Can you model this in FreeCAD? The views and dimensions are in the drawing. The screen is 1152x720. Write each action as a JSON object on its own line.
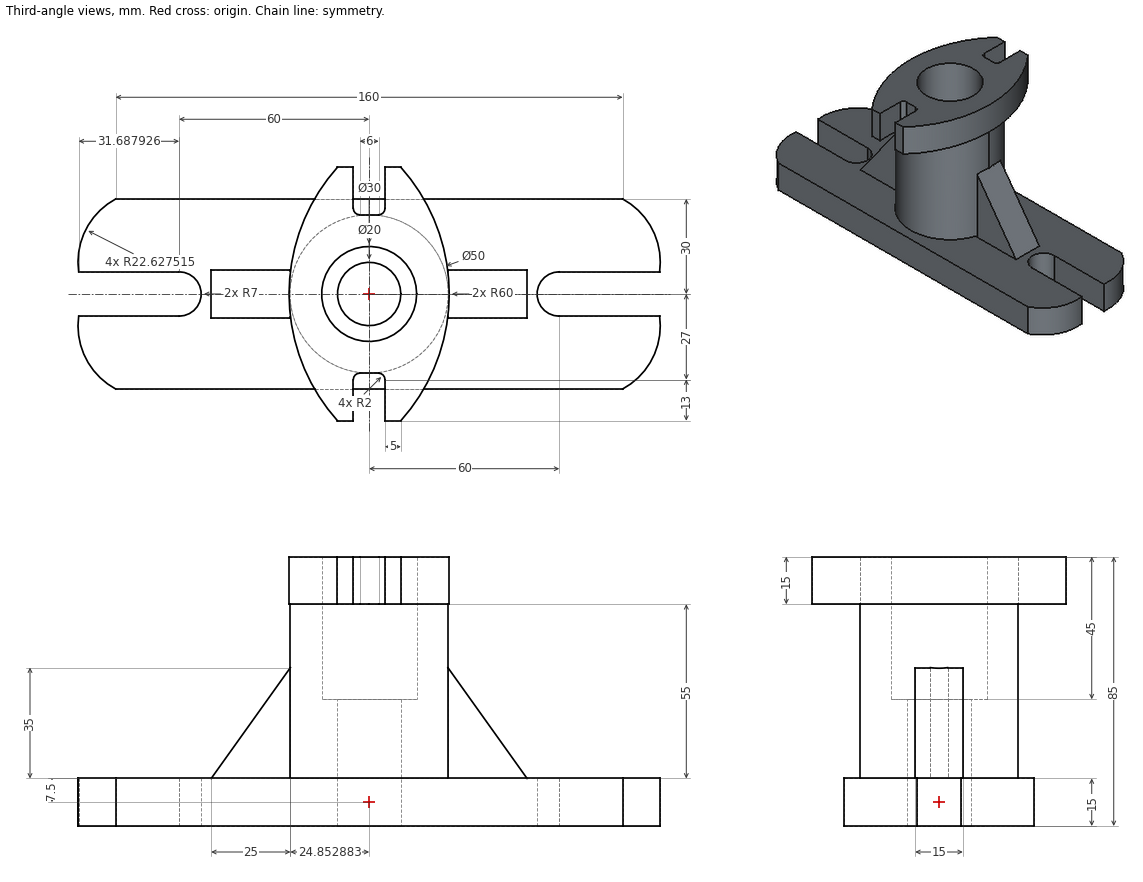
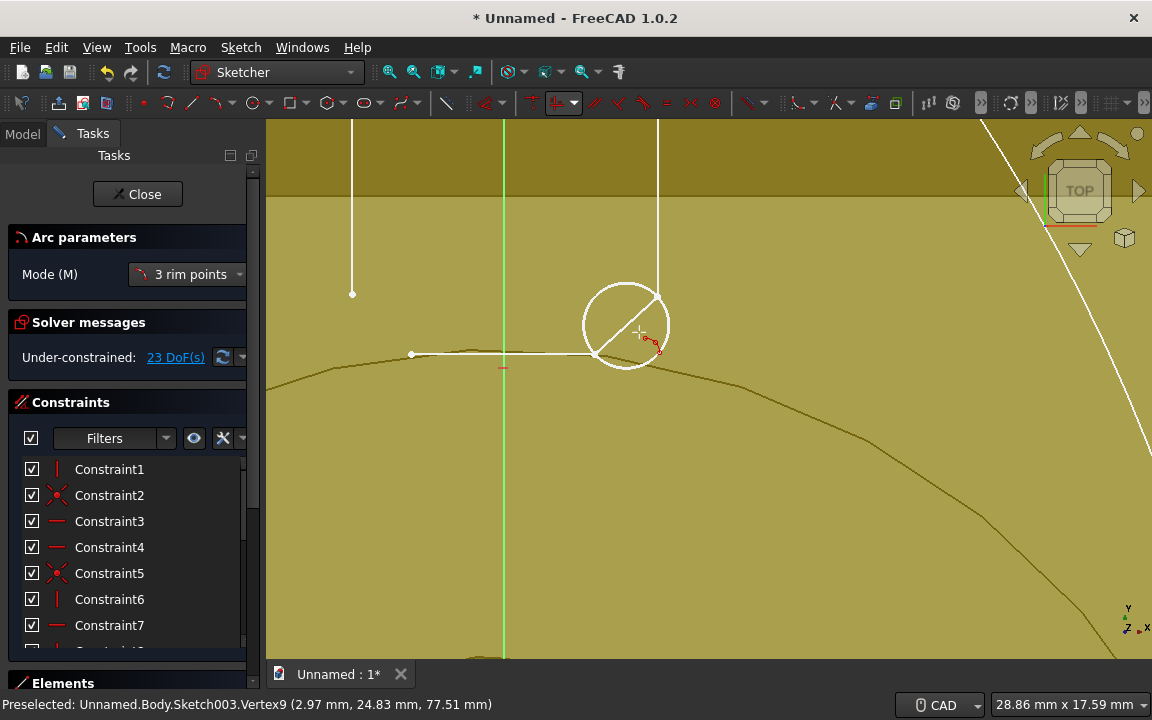
{"action": "left_click", "coordinate": [639, 331]}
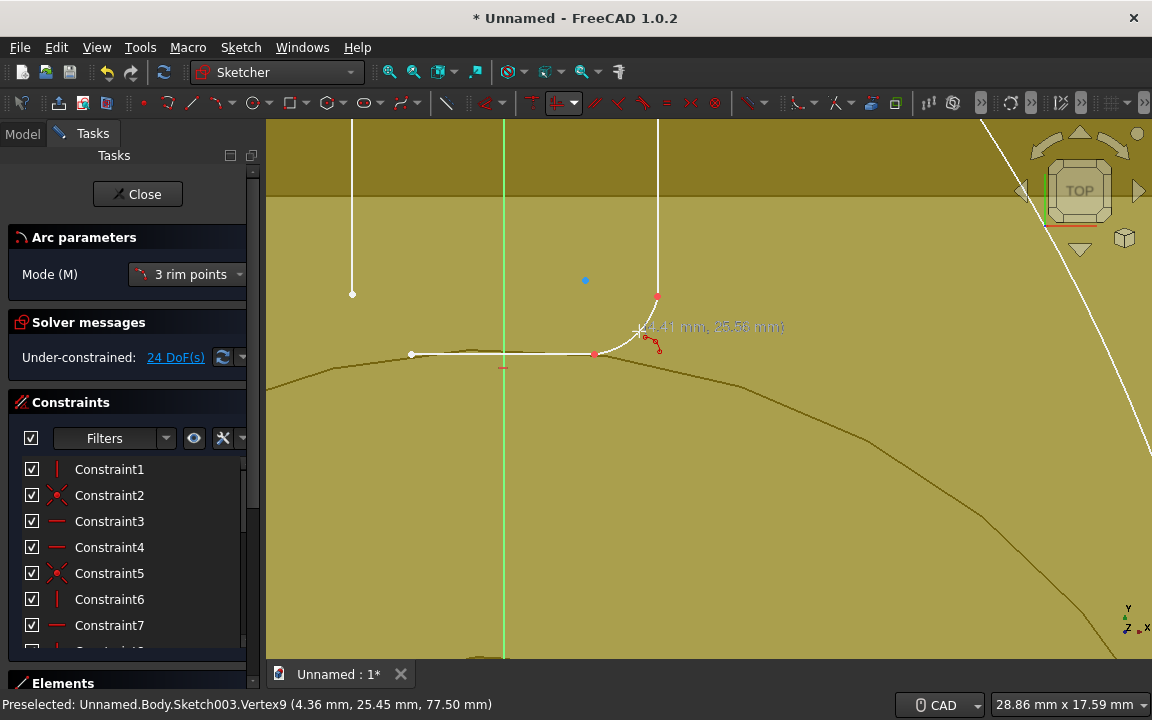
{"action": "scroll", "coordinate": [662, 275], "scroll_direction": "down", "scroll_amount": 10}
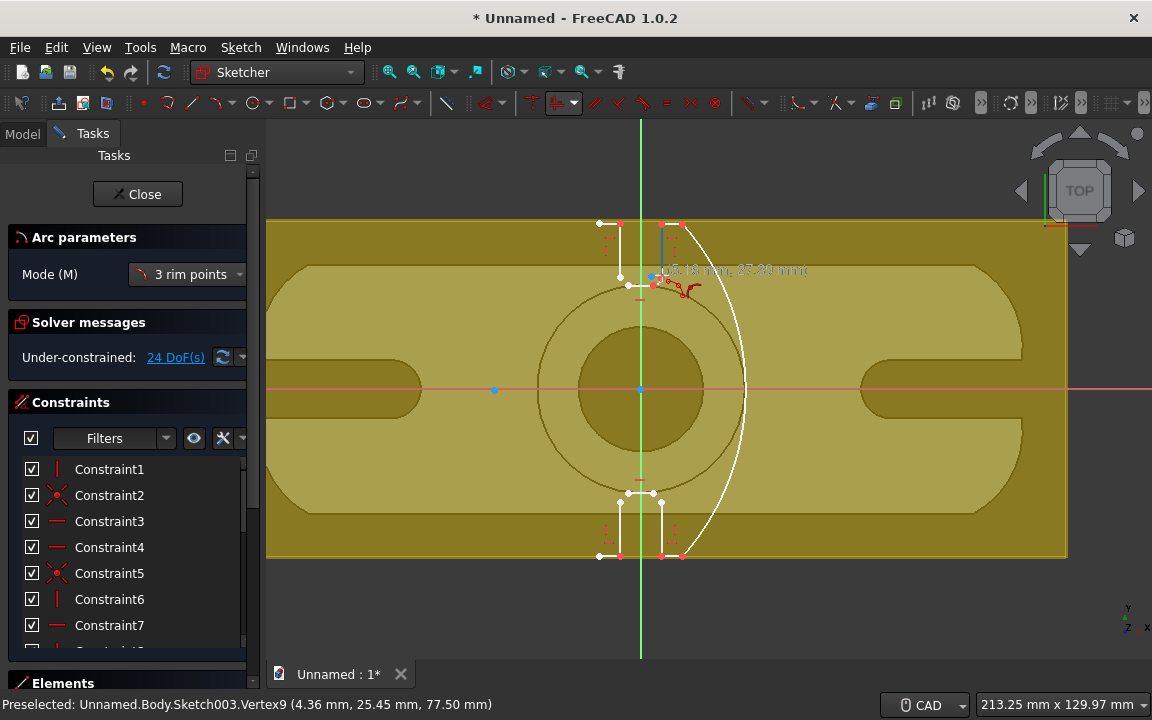
{"action": "scroll", "coordinate": [628, 285], "scroll_direction": "up", "scroll_amount": 2}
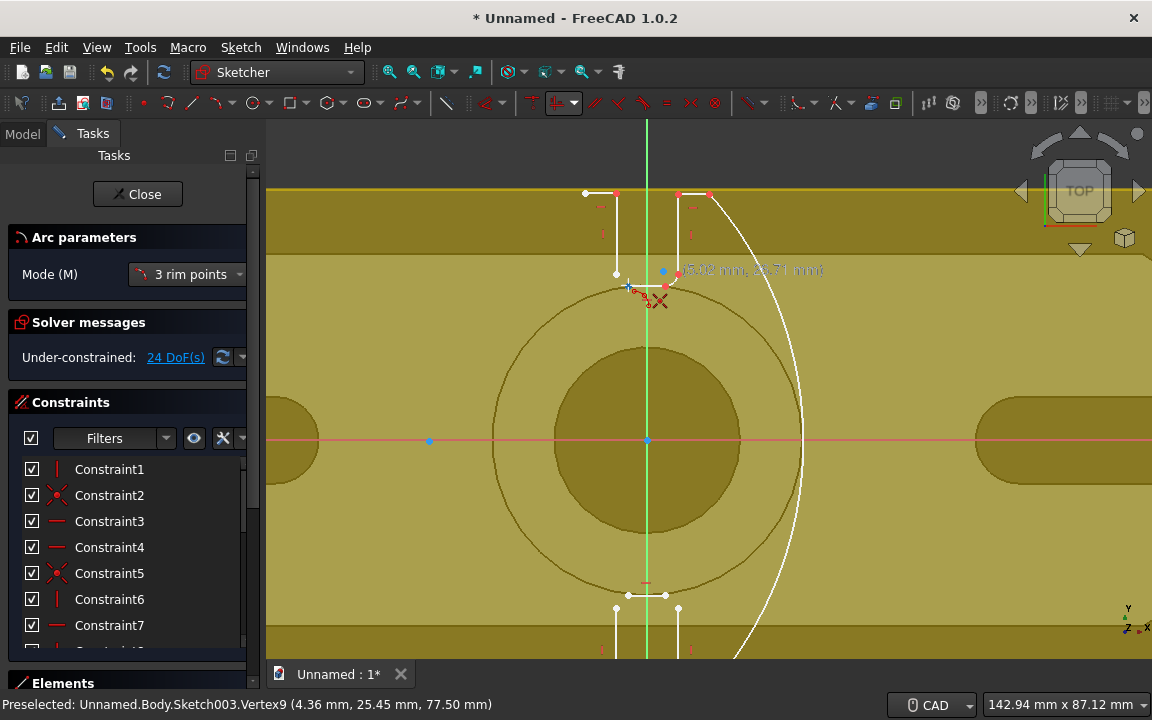
{"action": "left_click", "coordinate": [629, 286]}
{"action": "left_click", "coordinate": [617, 274]}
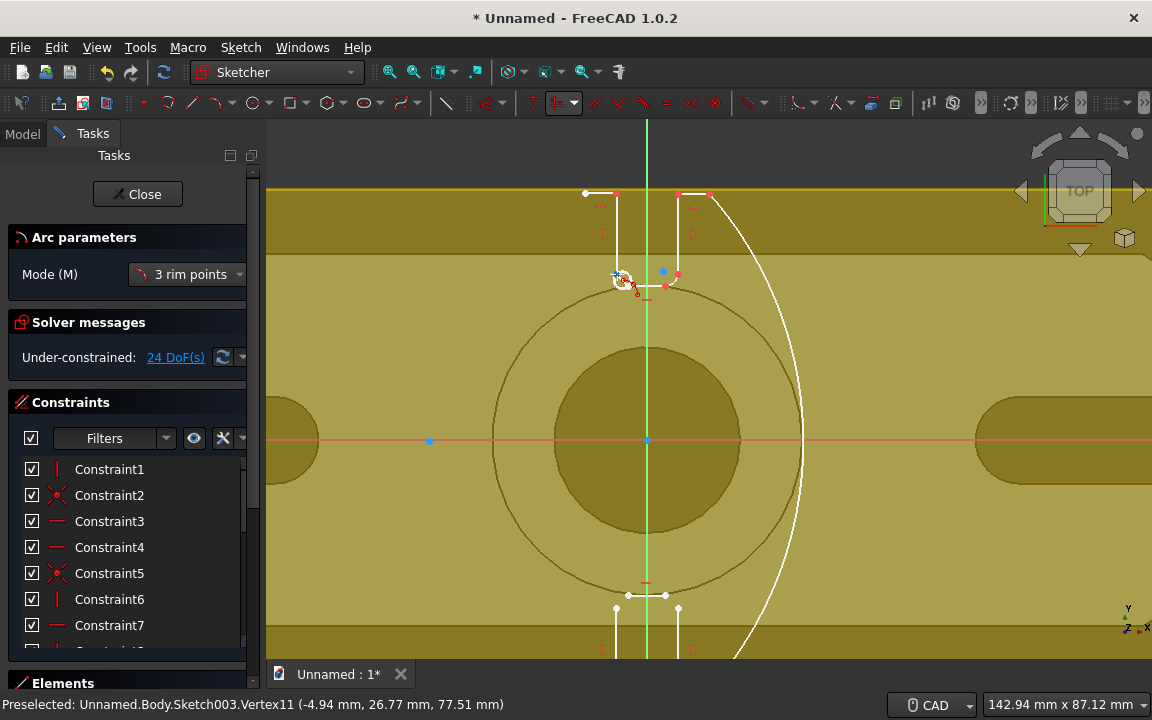
{"action": "scroll", "coordinate": [620, 282], "scroll_direction": "up", "scroll_amount": 8}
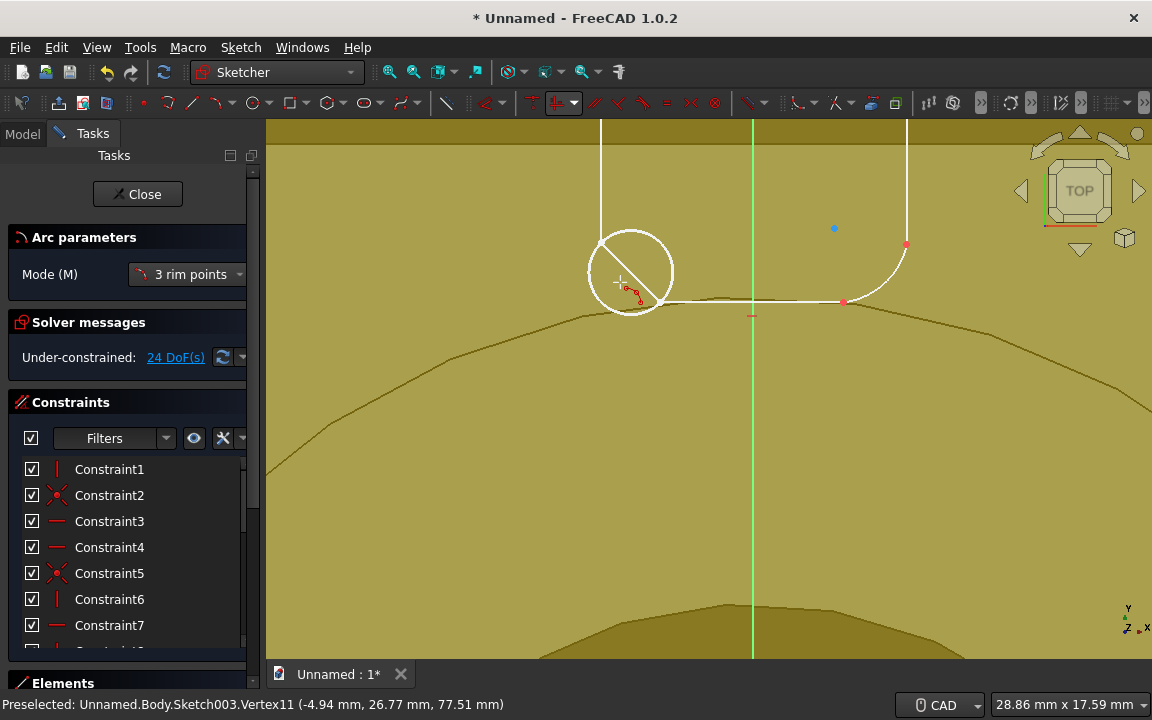
{"action": "left_click", "coordinate": [617, 279]}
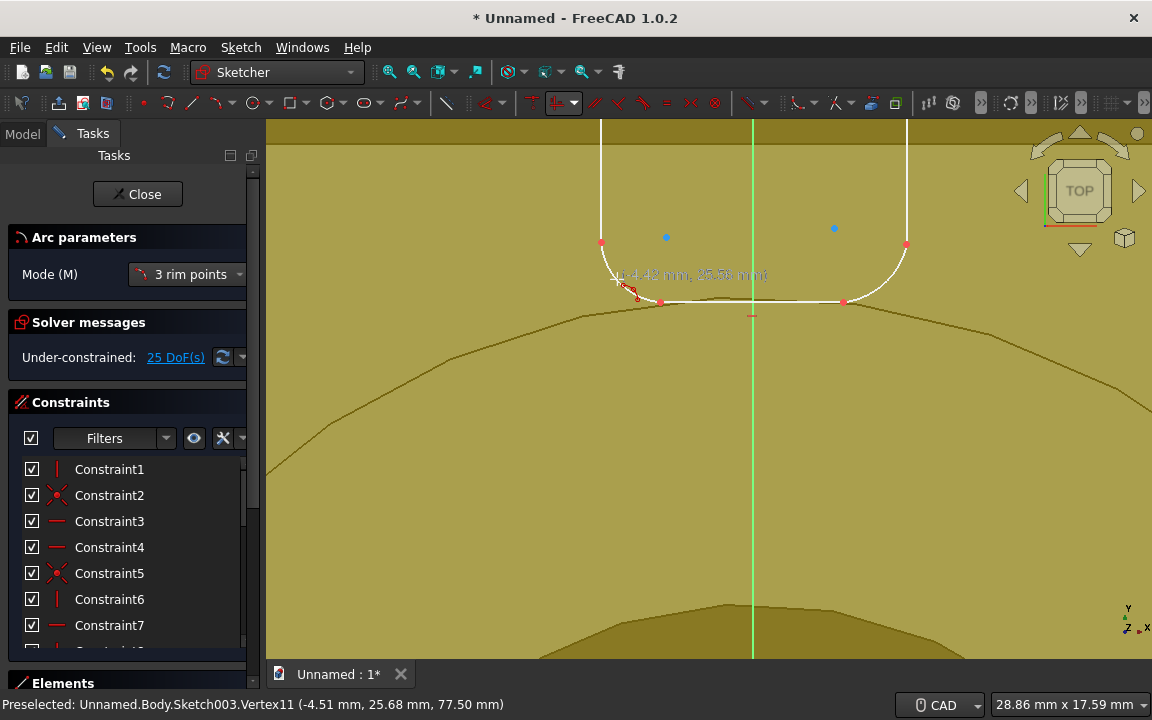
{"action": "scroll", "coordinate": [623, 283], "scroll_direction": "down", "scroll_amount": 10}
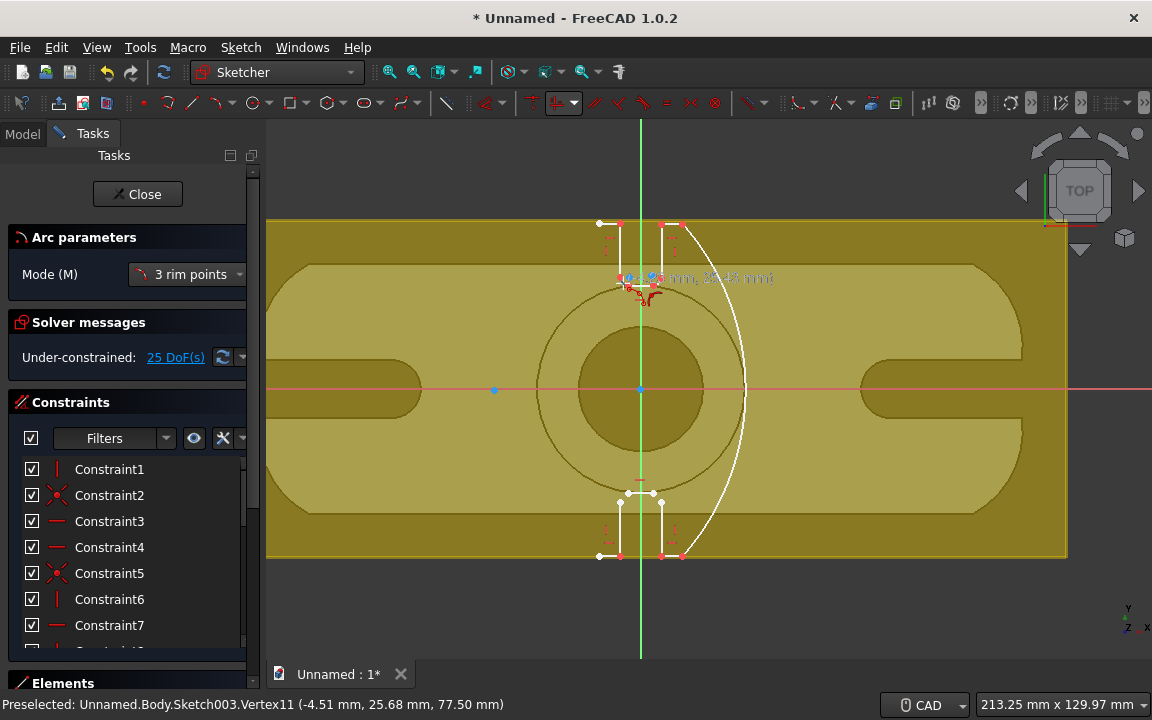
{"action": "scroll", "coordinate": [599, 223], "scroll_direction": "up", "scroll_amount": 3}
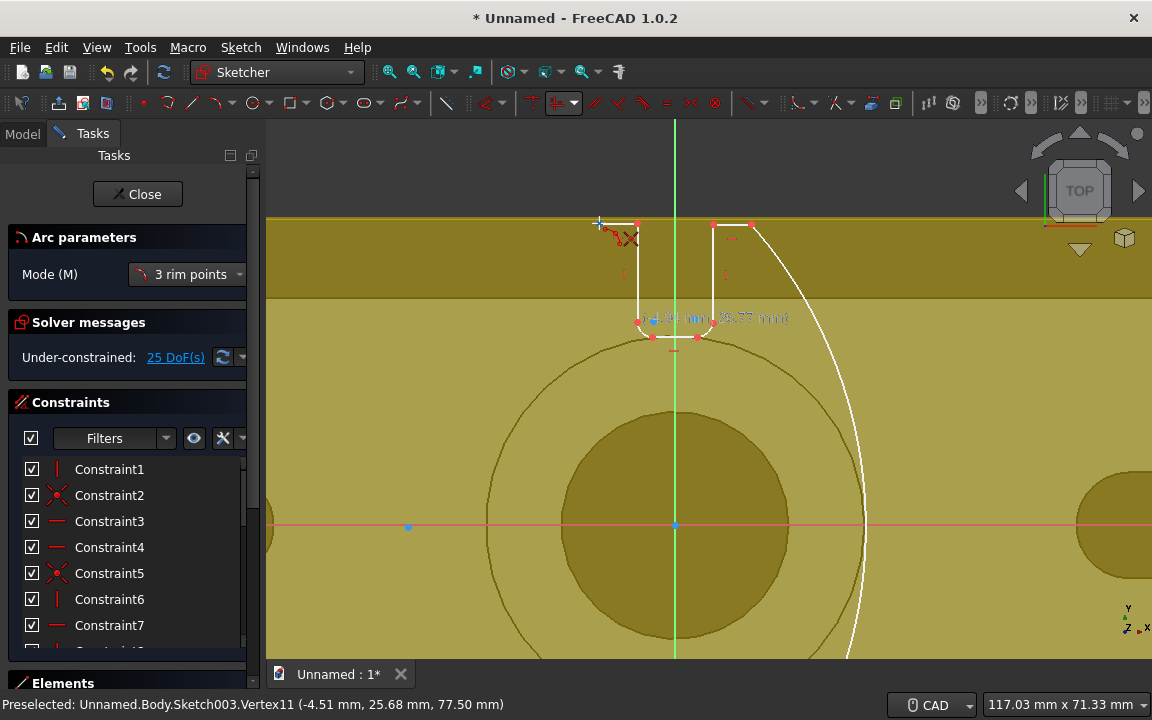
{"action": "left_click", "coordinate": [600, 224]}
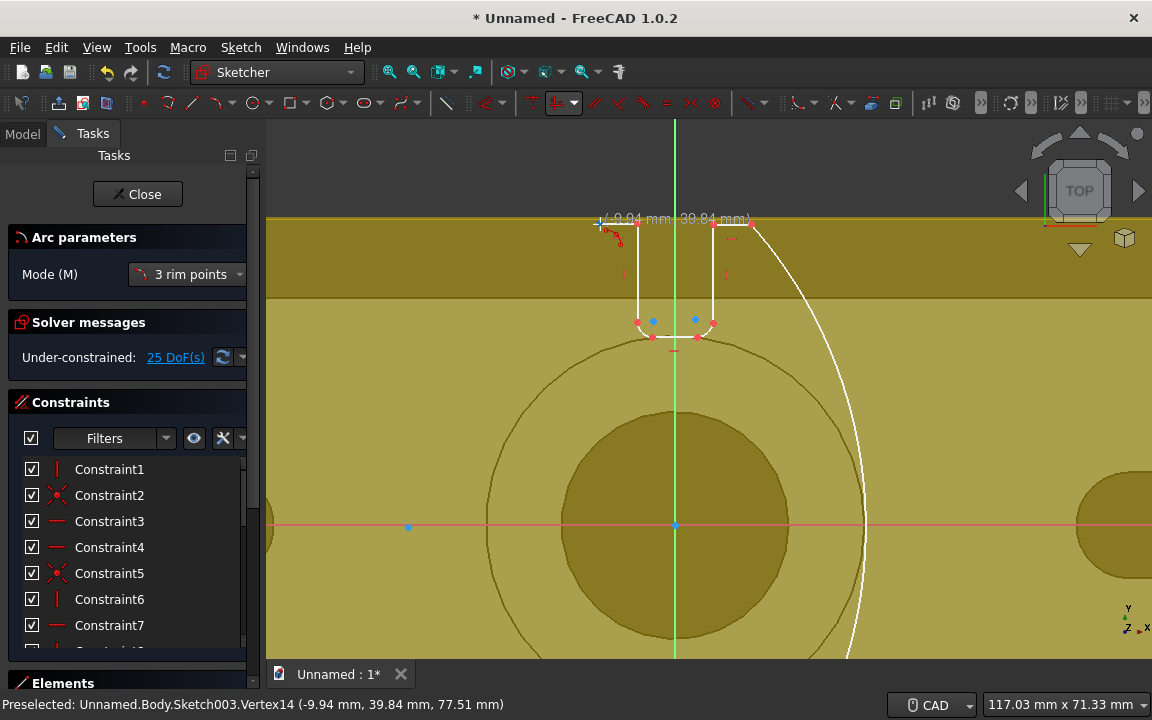
{"action": "scroll", "coordinate": [598, 223], "scroll_direction": "down", "scroll_amount": 3}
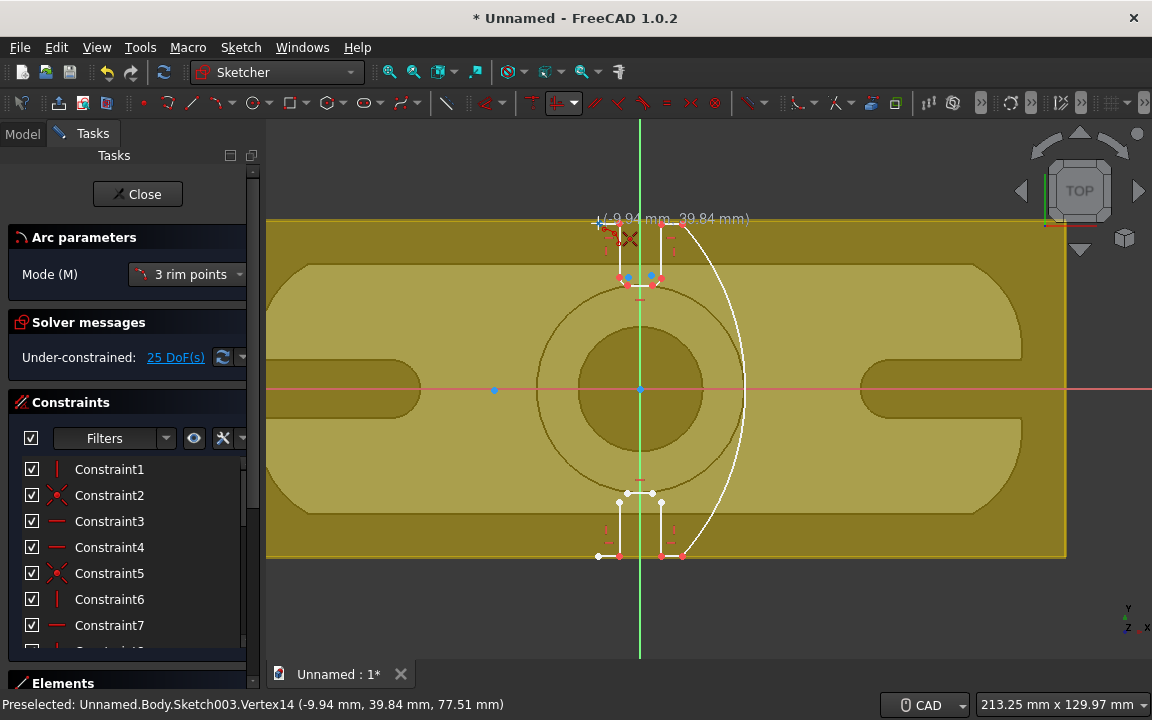
{"action": "scroll", "coordinate": [599, 555], "scroll_direction": "up", "scroll_amount": 3}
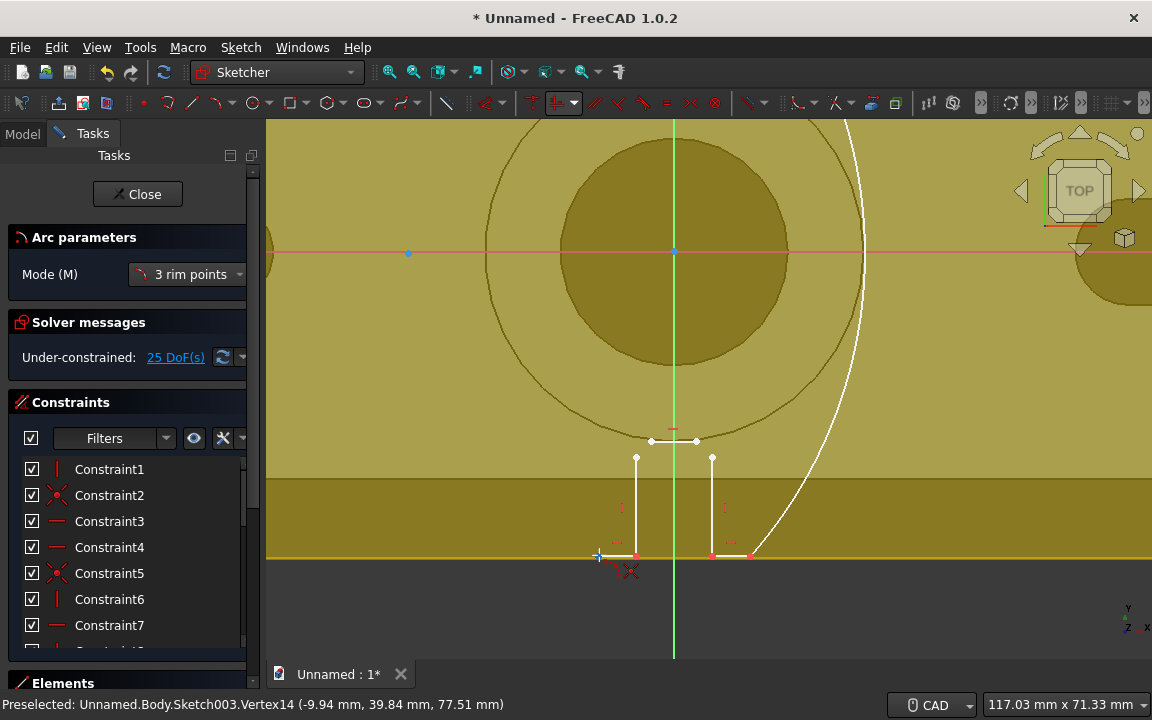
{"action": "left_click", "coordinate": [598, 556]}
{"action": "left_click", "coordinate": [488, 186]}